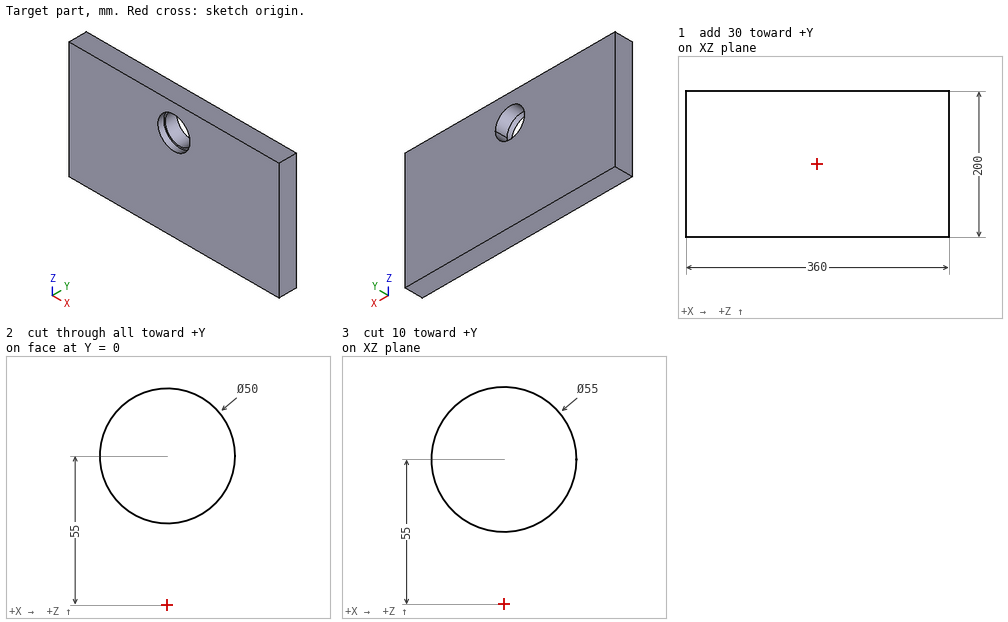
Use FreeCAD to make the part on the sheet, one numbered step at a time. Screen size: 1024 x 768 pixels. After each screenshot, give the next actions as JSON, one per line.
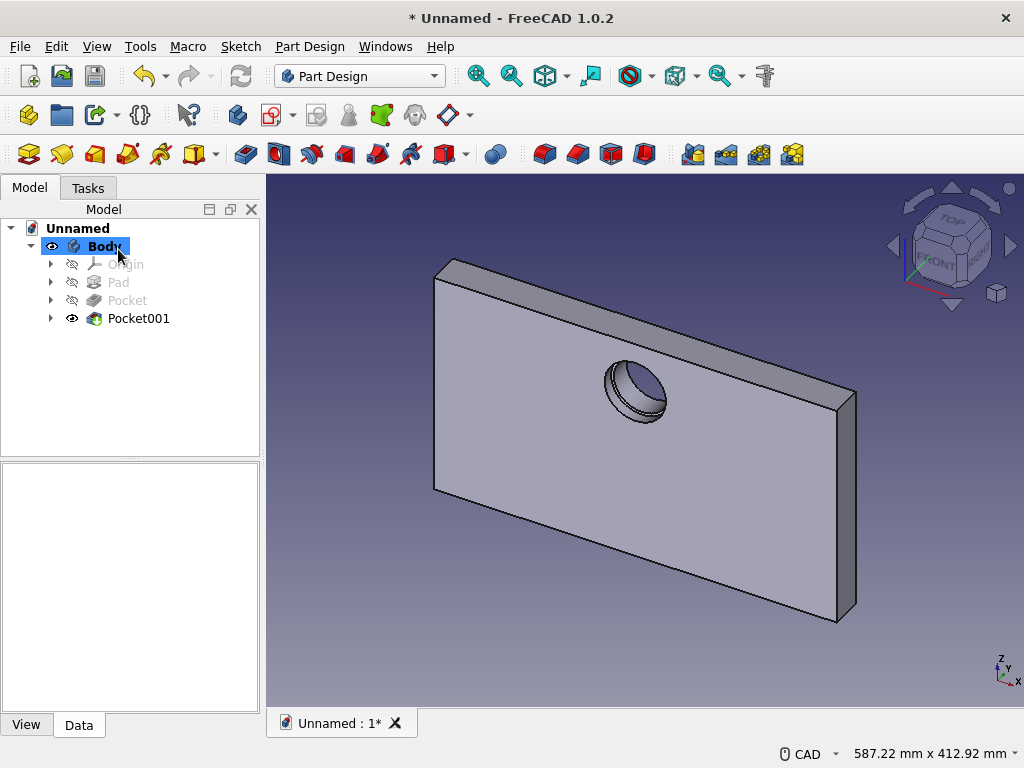
{"action": "key", "text": "0"}